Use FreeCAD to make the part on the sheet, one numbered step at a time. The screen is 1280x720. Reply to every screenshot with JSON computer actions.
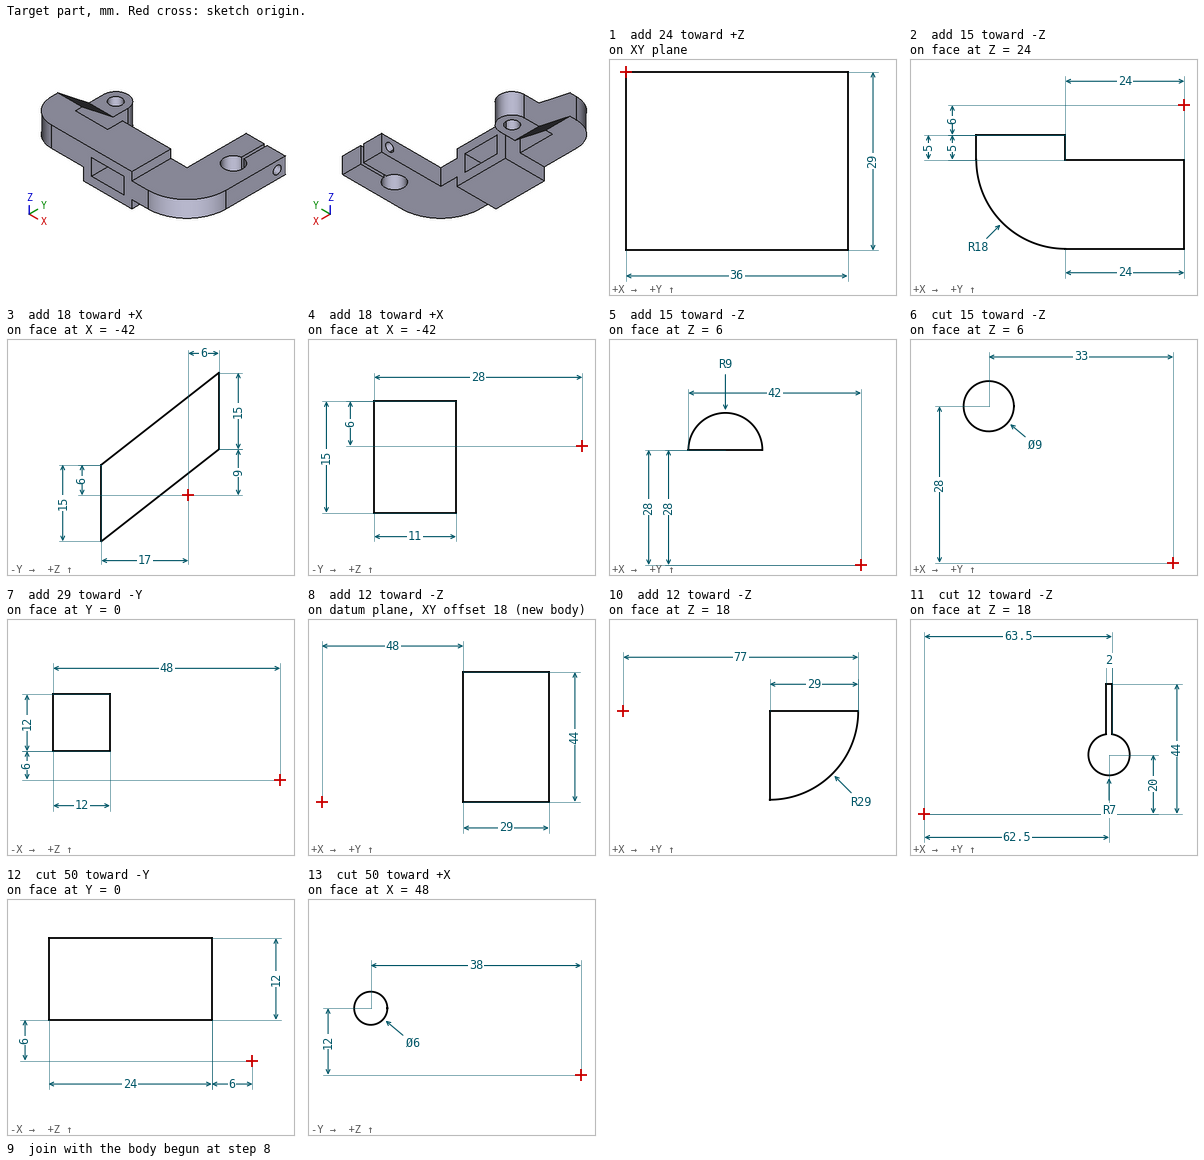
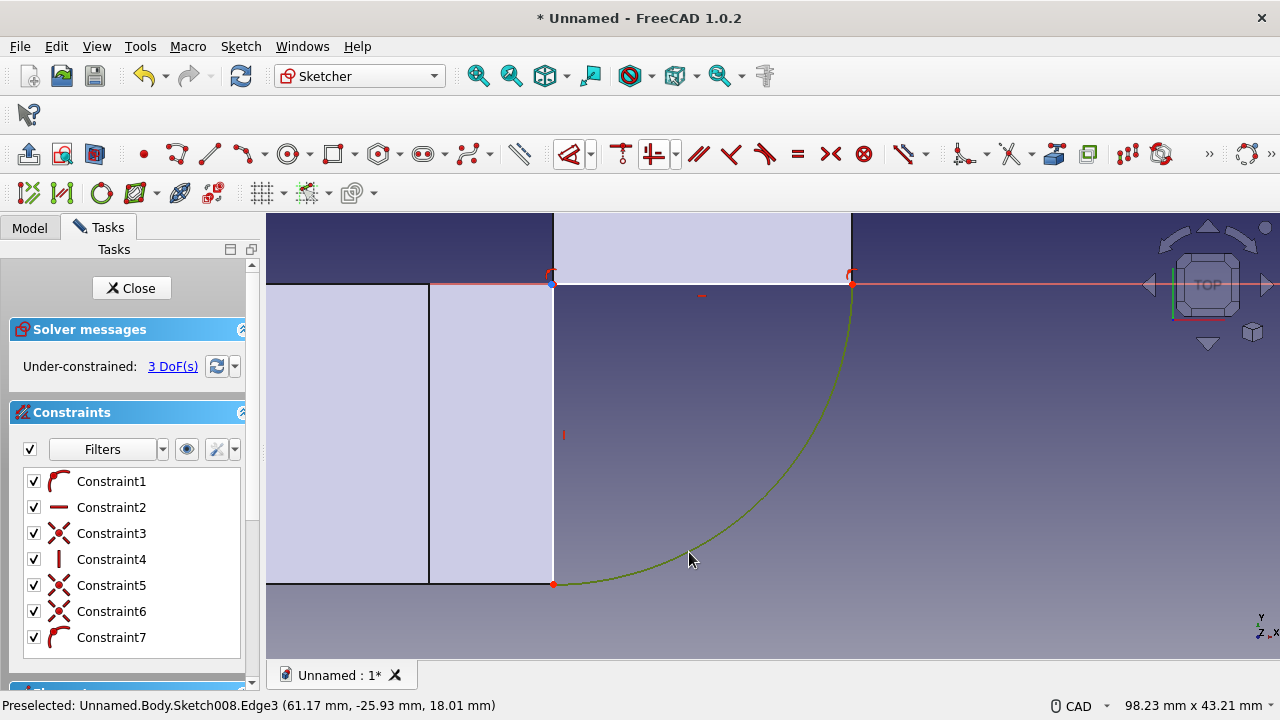
{"action": "left_click", "coordinate": [590, 154]}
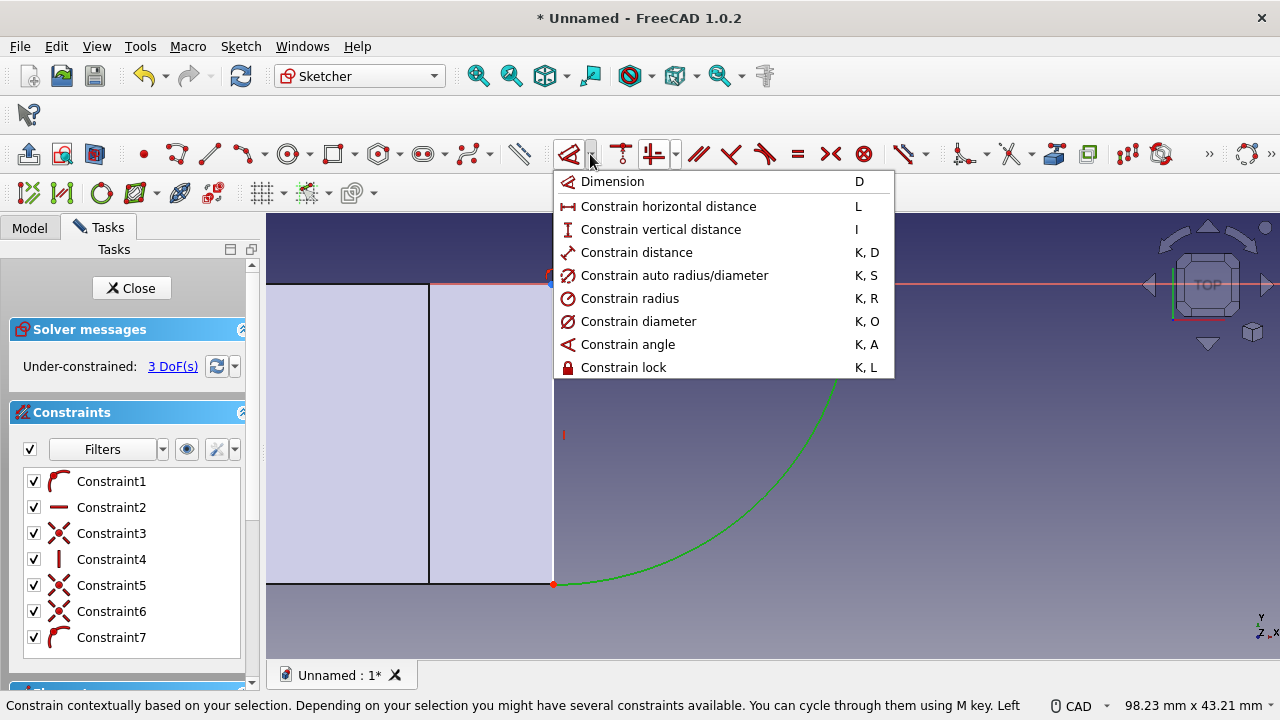
{"action": "left_click", "coordinate": [724, 298]}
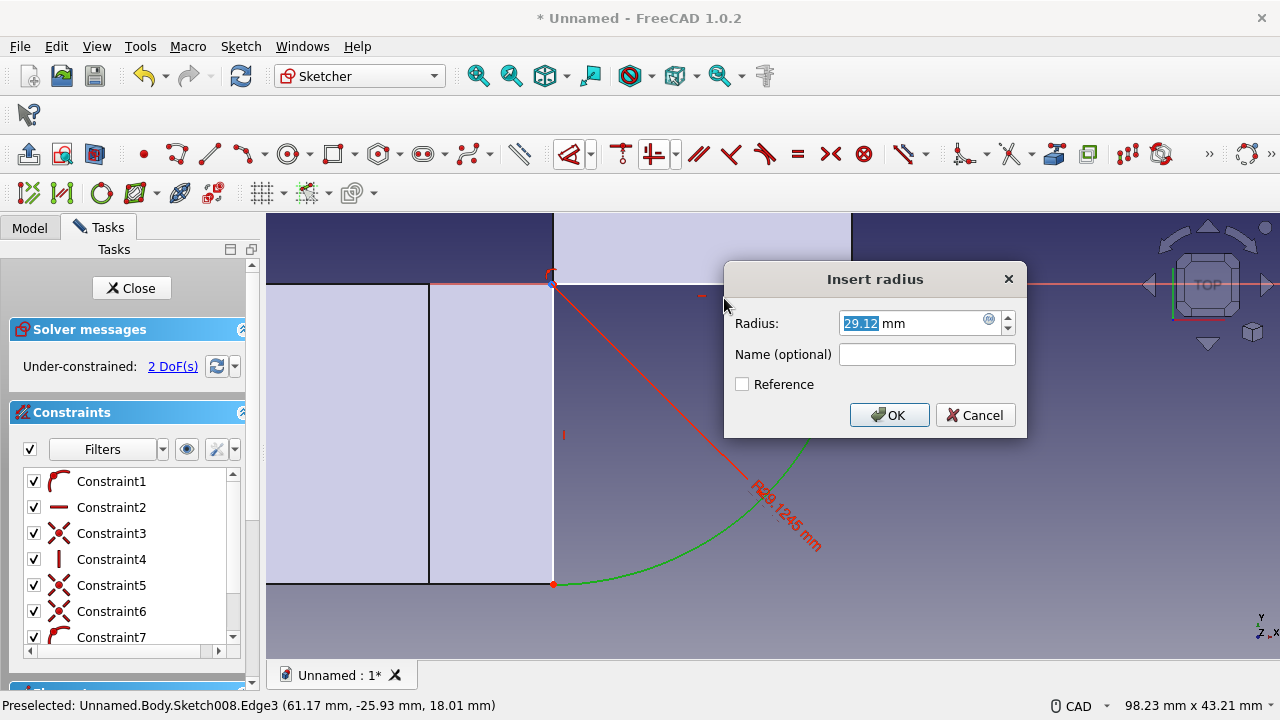
{"action": "type", "text": "29"}
{"action": "key", "text": "Return"}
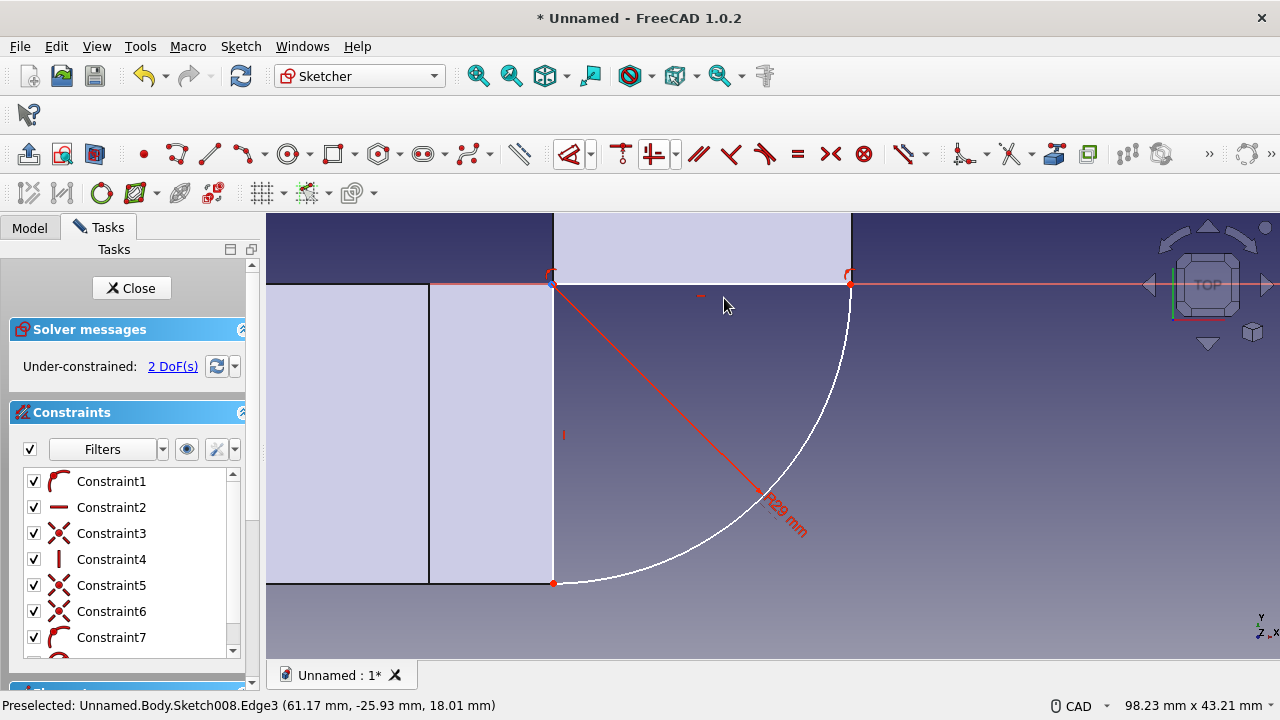
{"action": "left_click", "coordinate": [762, 284]}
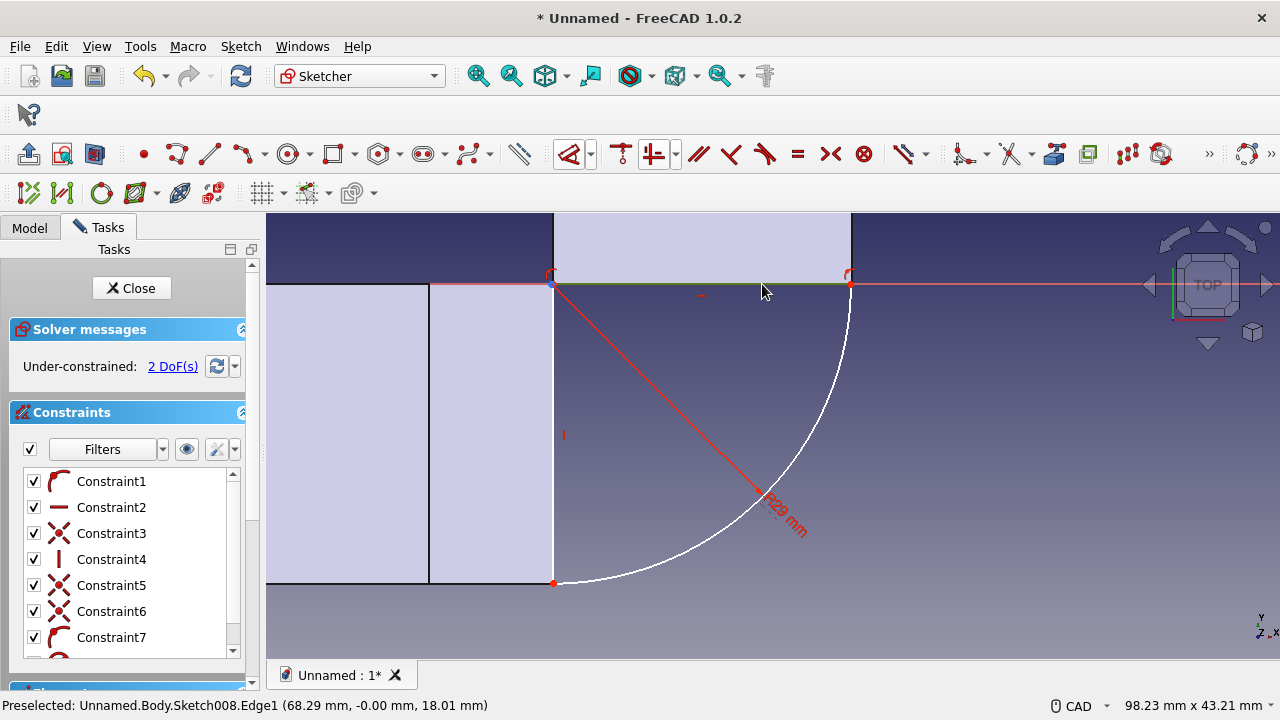
{"action": "key", "text": "l"}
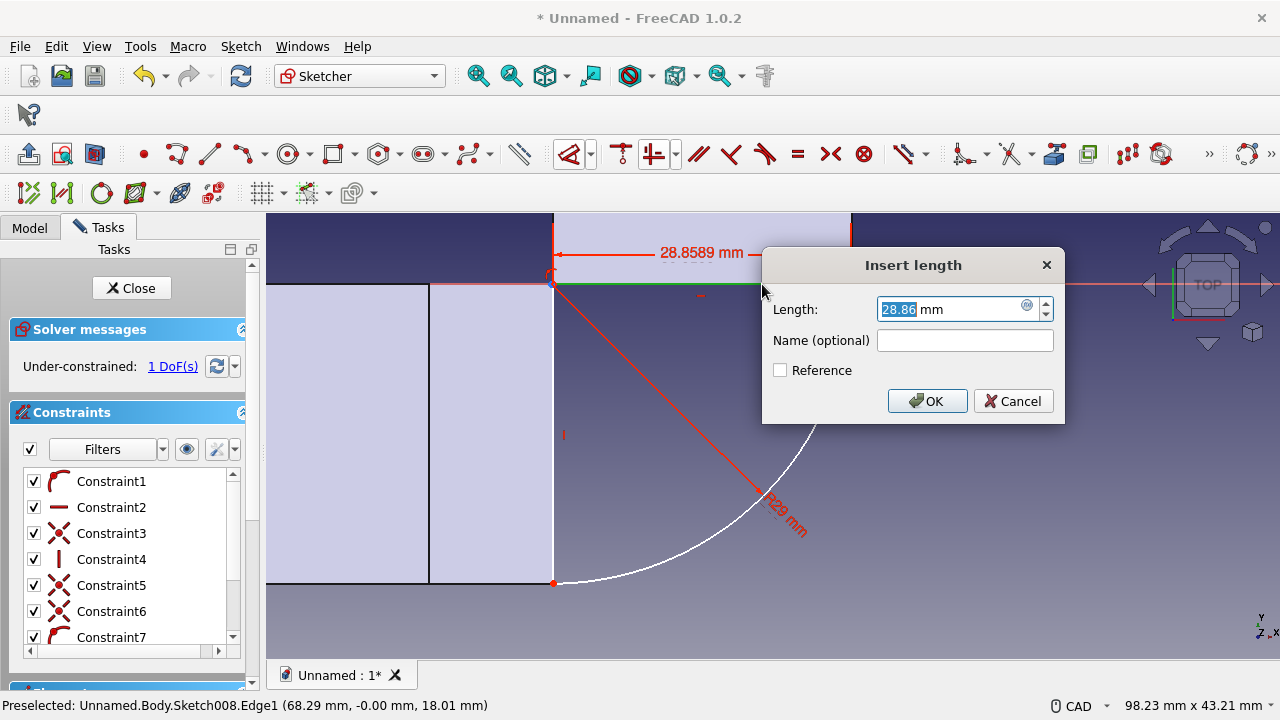
{"action": "type", "text": "29"}
{"action": "key", "text": "Return"}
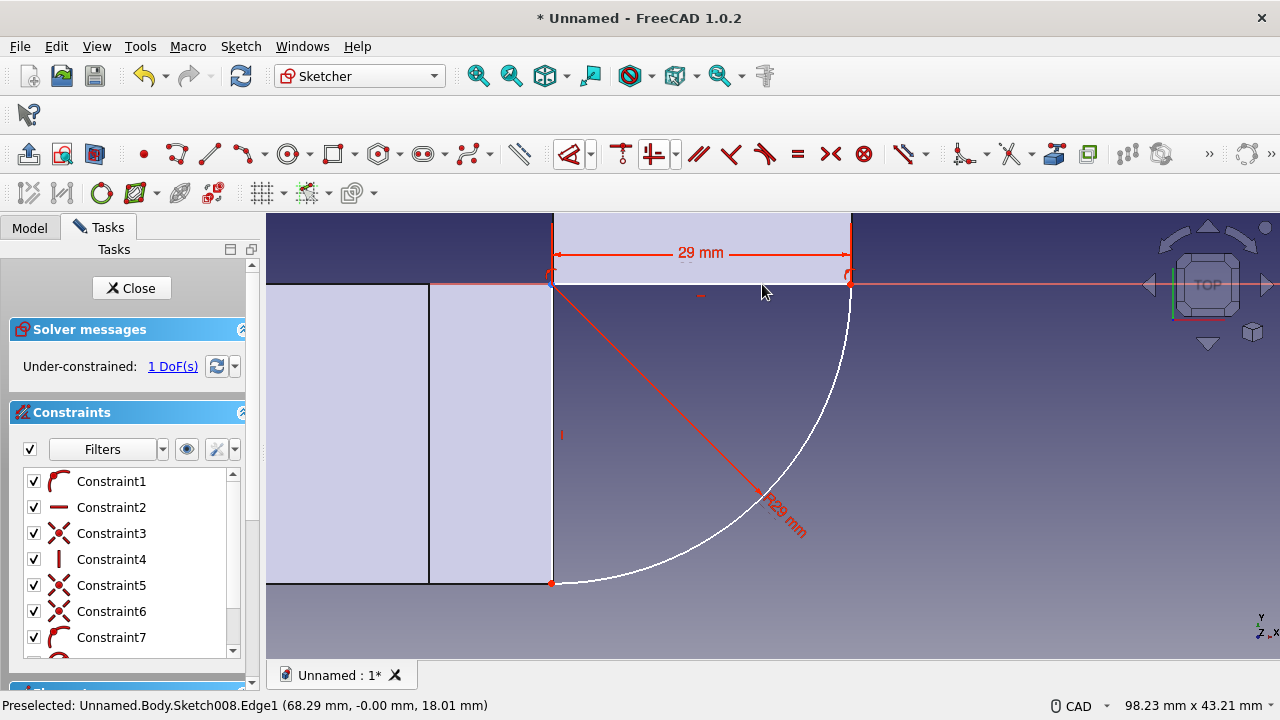
{"action": "left_click", "coordinate": [851, 284]}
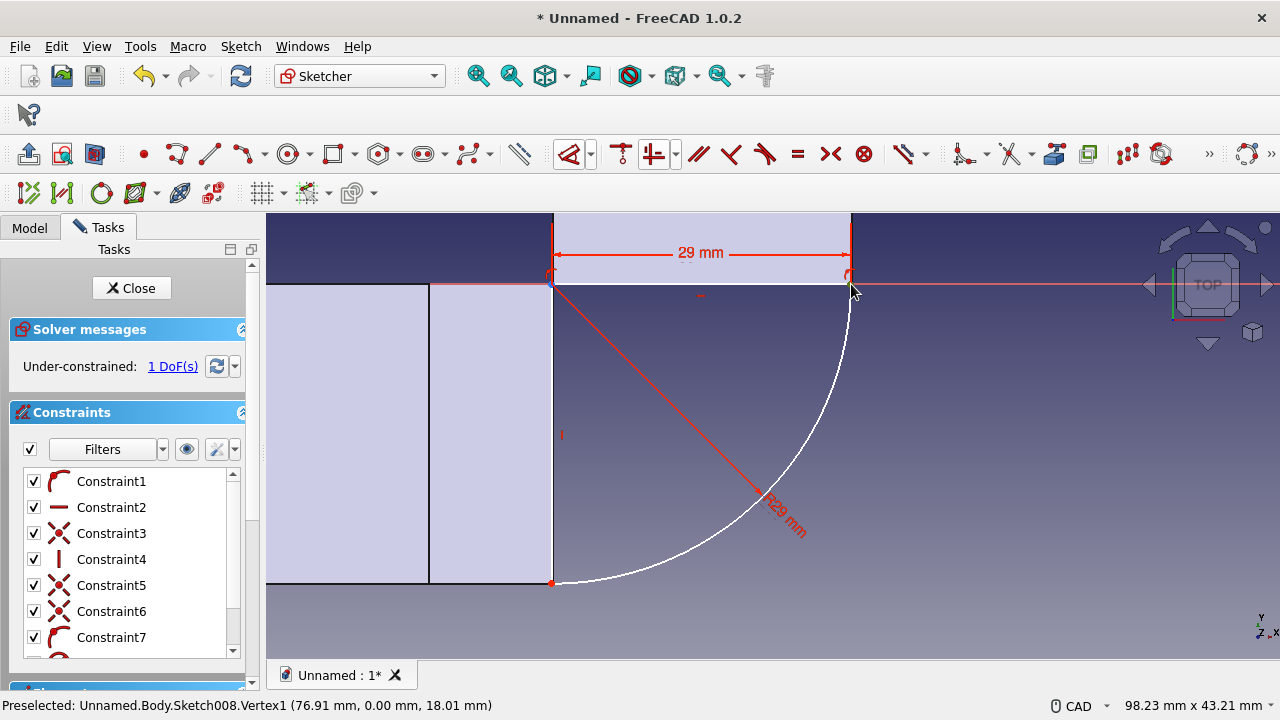
{"action": "left_click", "coordinate": [590, 154]}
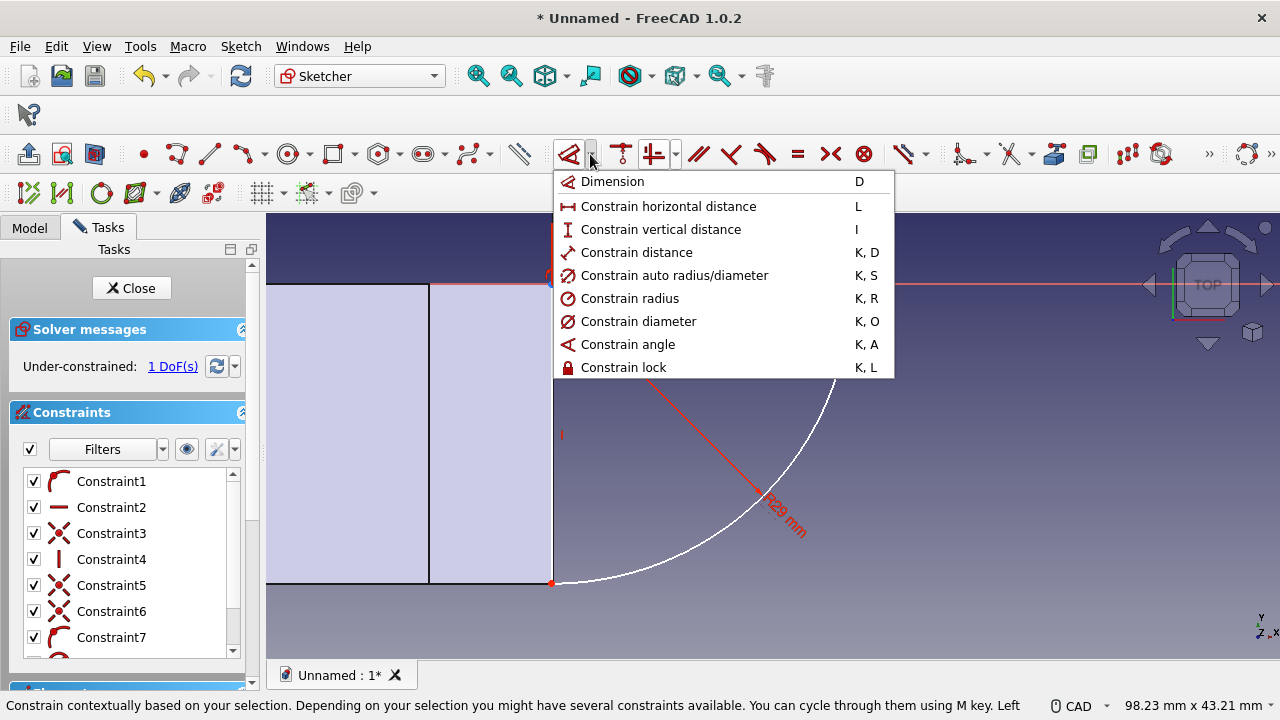
{"action": "left_click", "coordinate": [724, 206]}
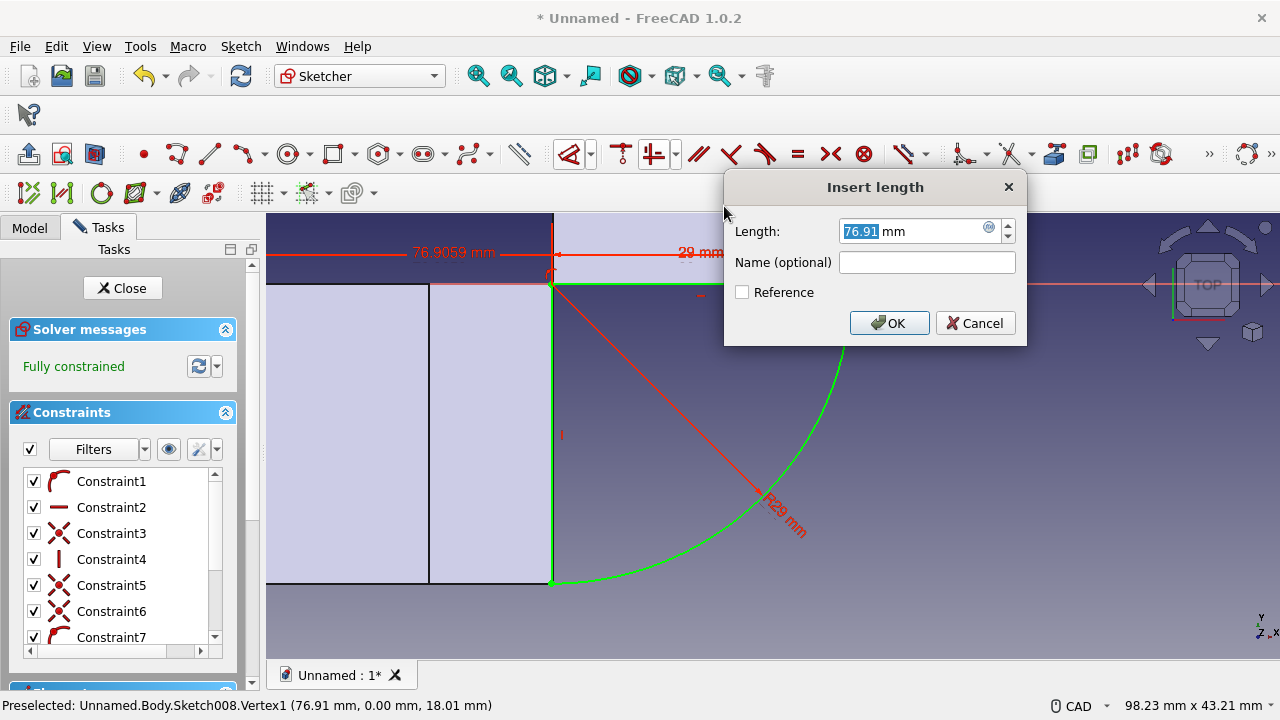
{"action": "type", "text": "77"}
{"action": "key", "text": "Return"}